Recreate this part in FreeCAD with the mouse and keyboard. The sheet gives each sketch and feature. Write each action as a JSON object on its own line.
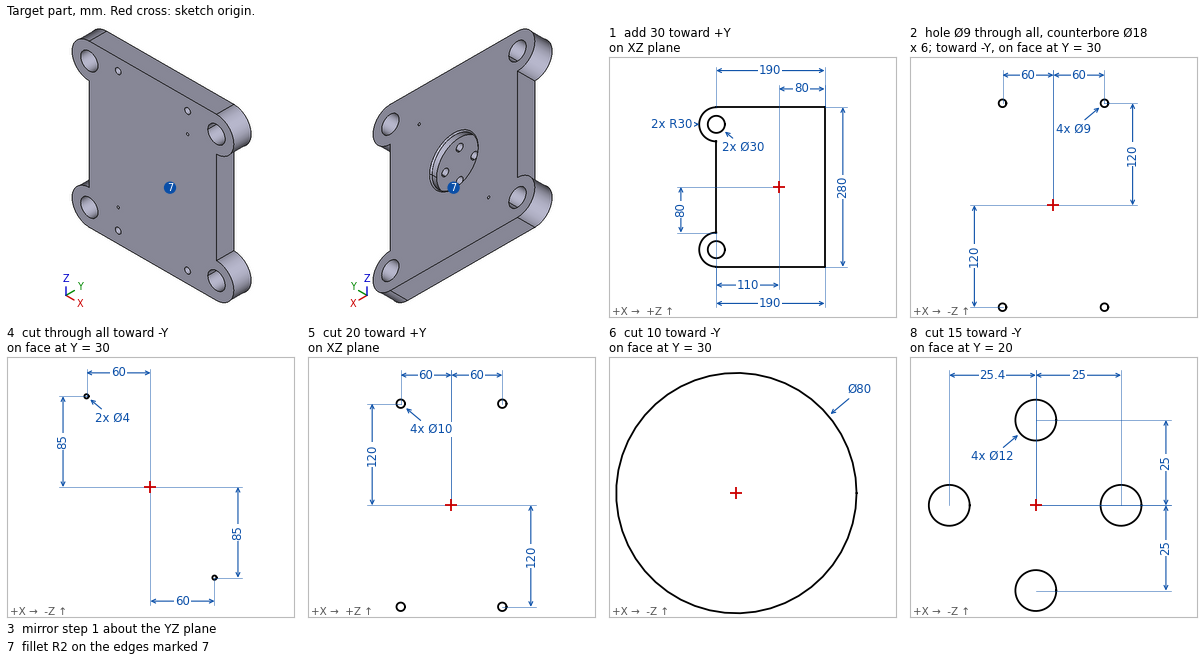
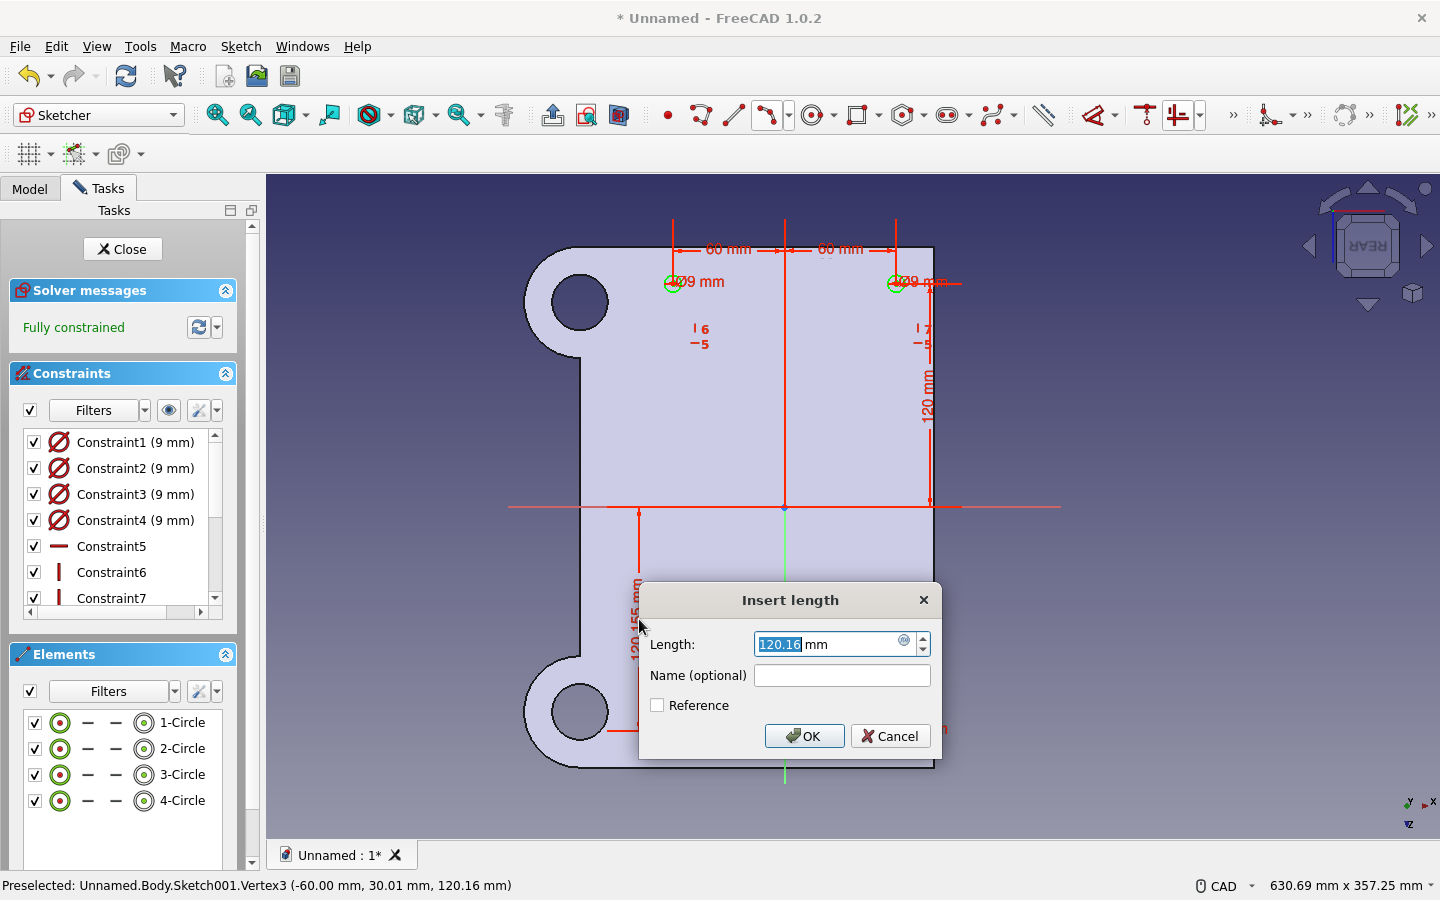
{"action": "type", "text": "120"}
{"action": "key", "text": "Return"}
{"action": "key", "text": "Escape"}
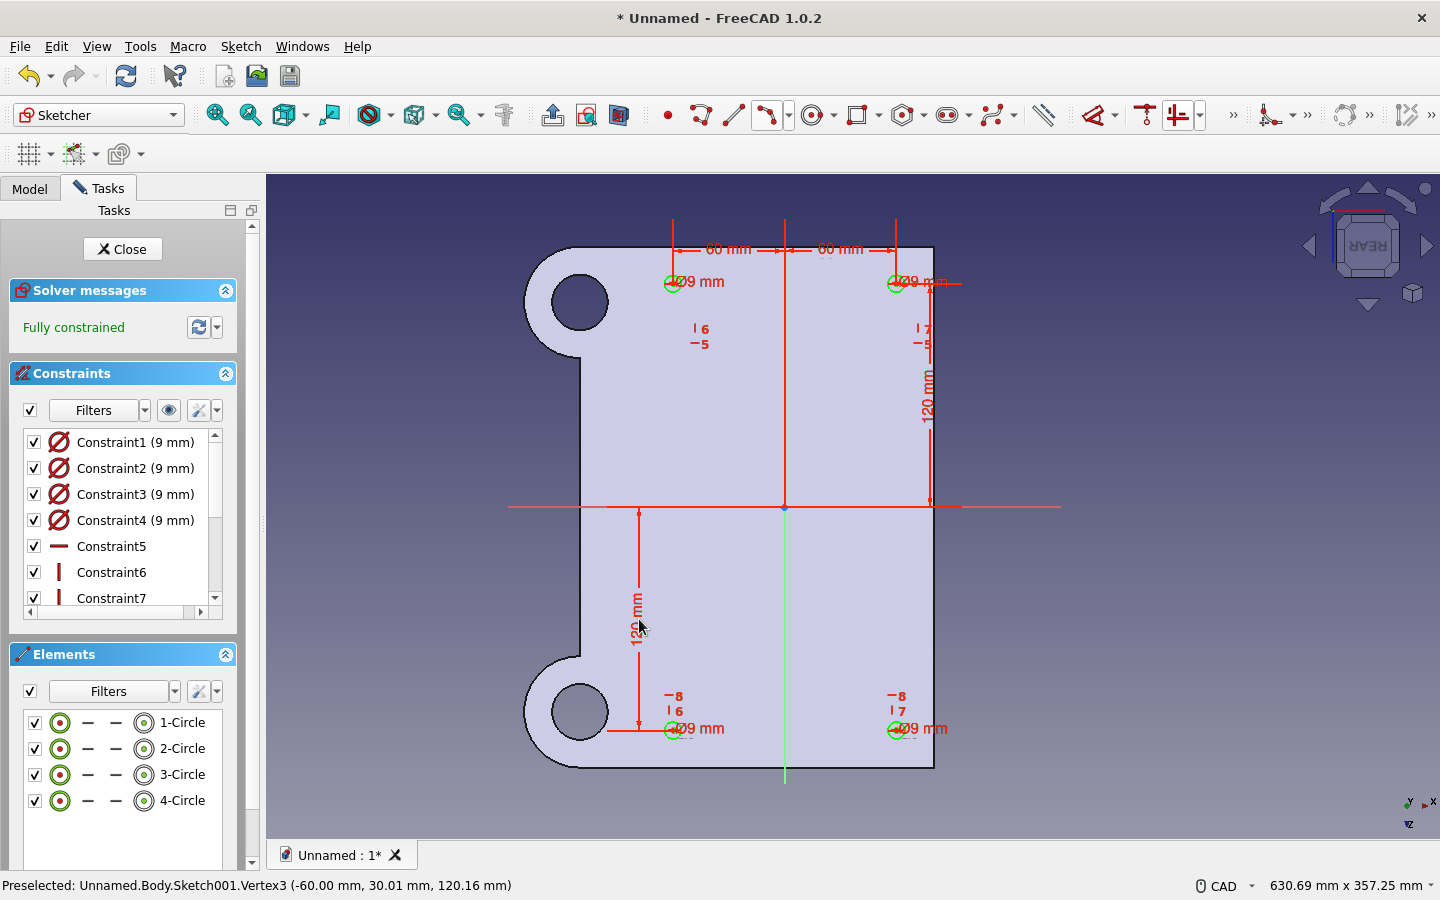
{"action": "left_click", "coordinate": [123, 249]}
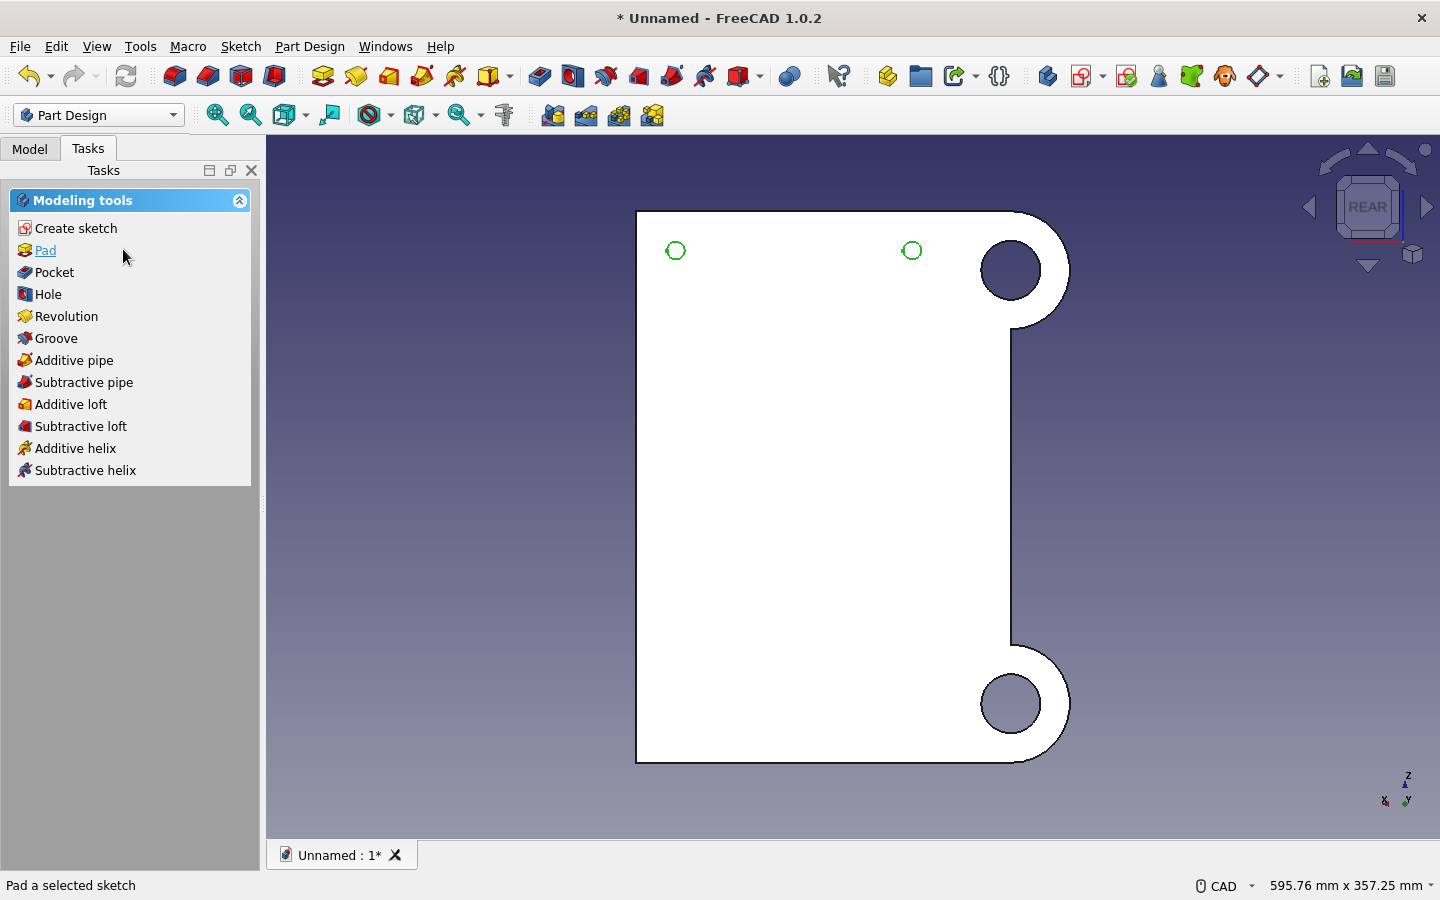
{"action": "left_click", "coordinate": [573, 76]}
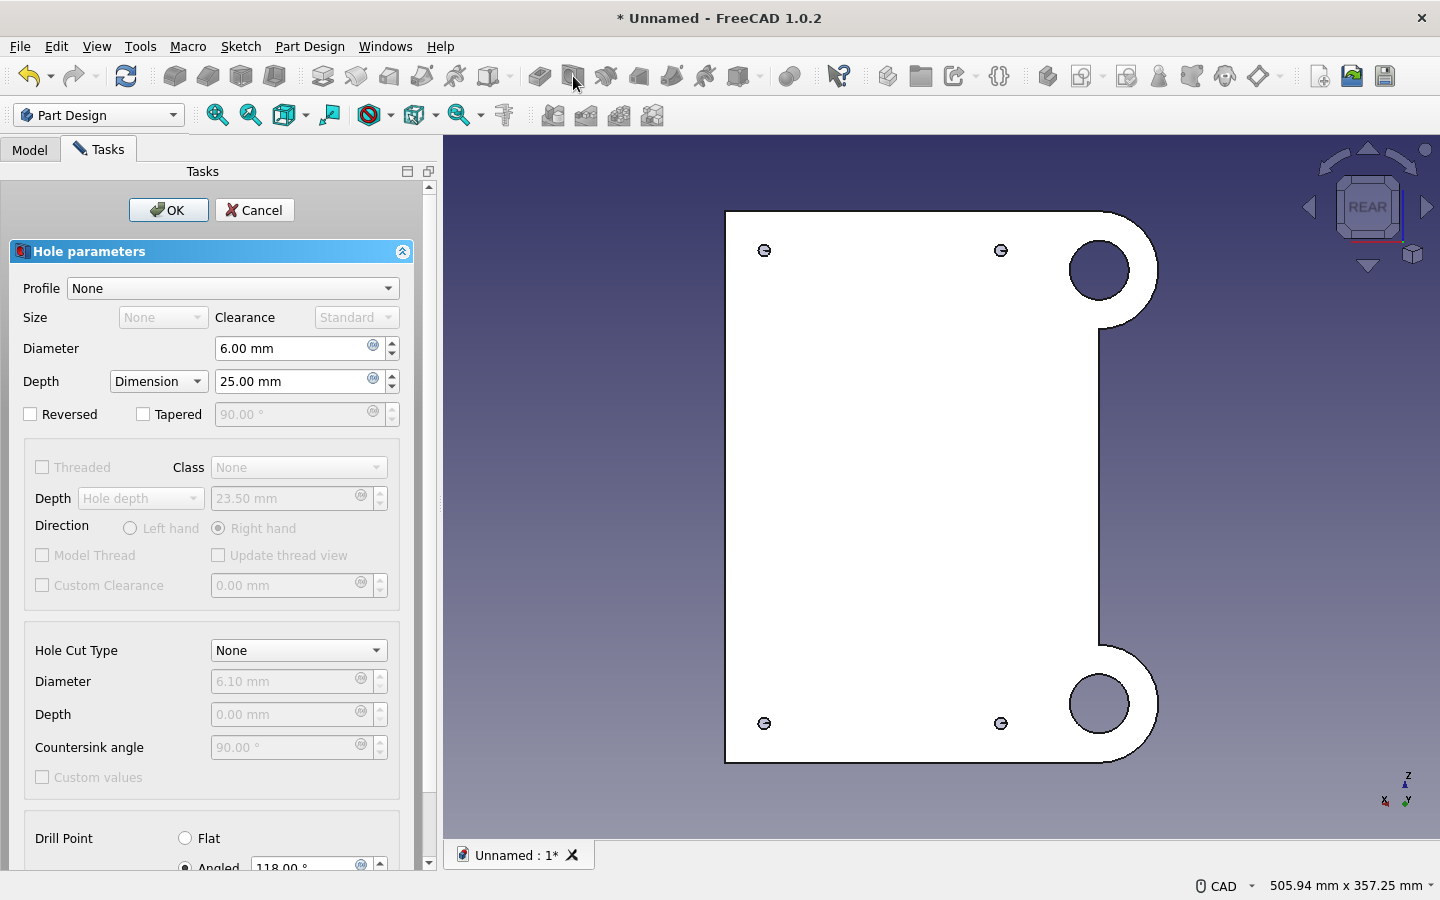
{"action": "triple_click", "coordinate": [300, 348]}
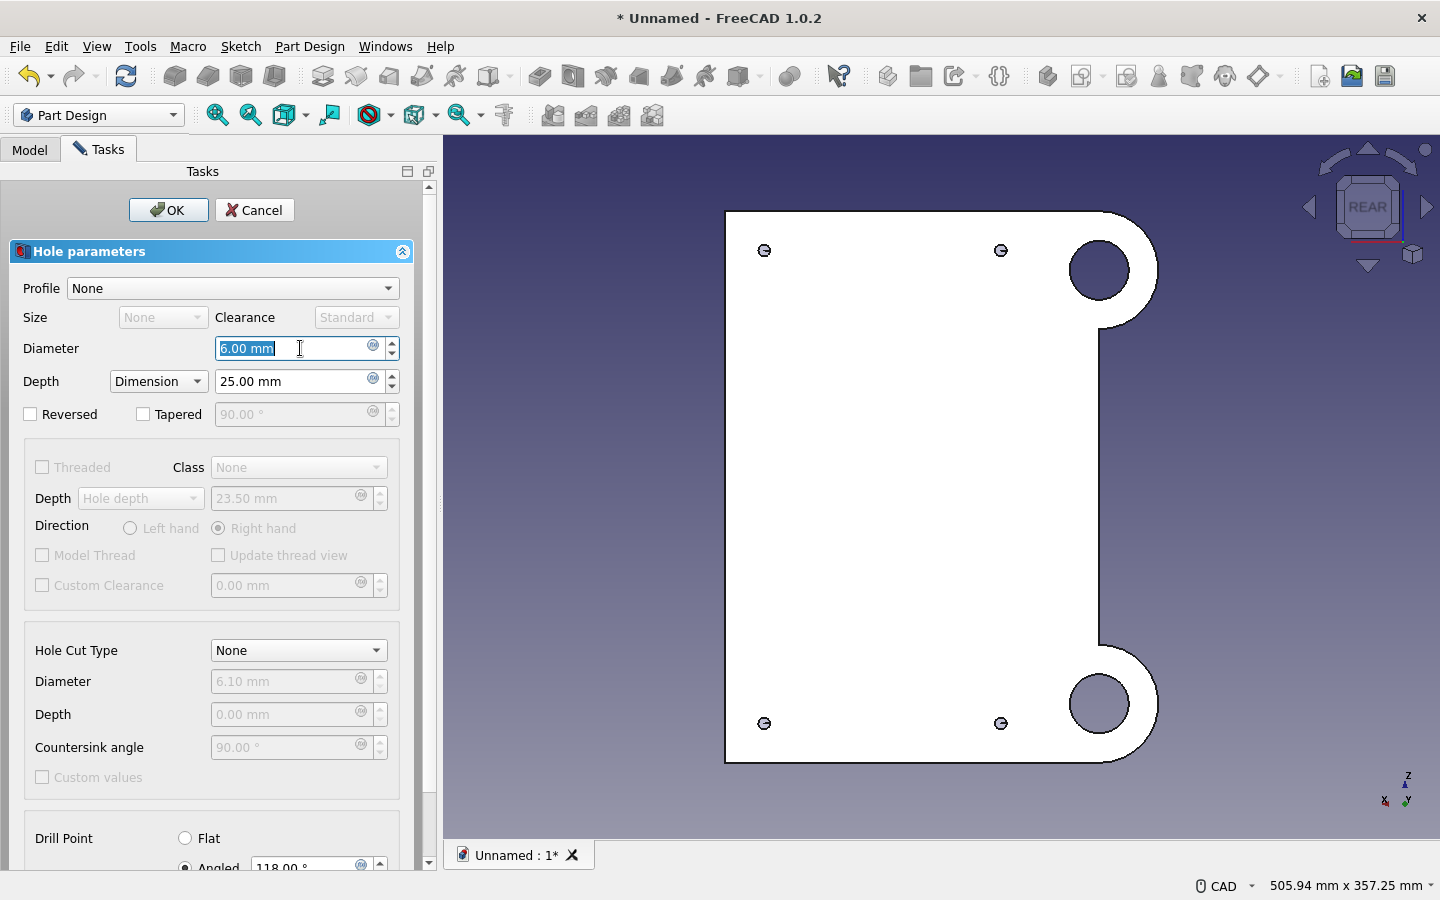
{"action": "type", "text": "9"}
{"action": "key", "text": "Tab"}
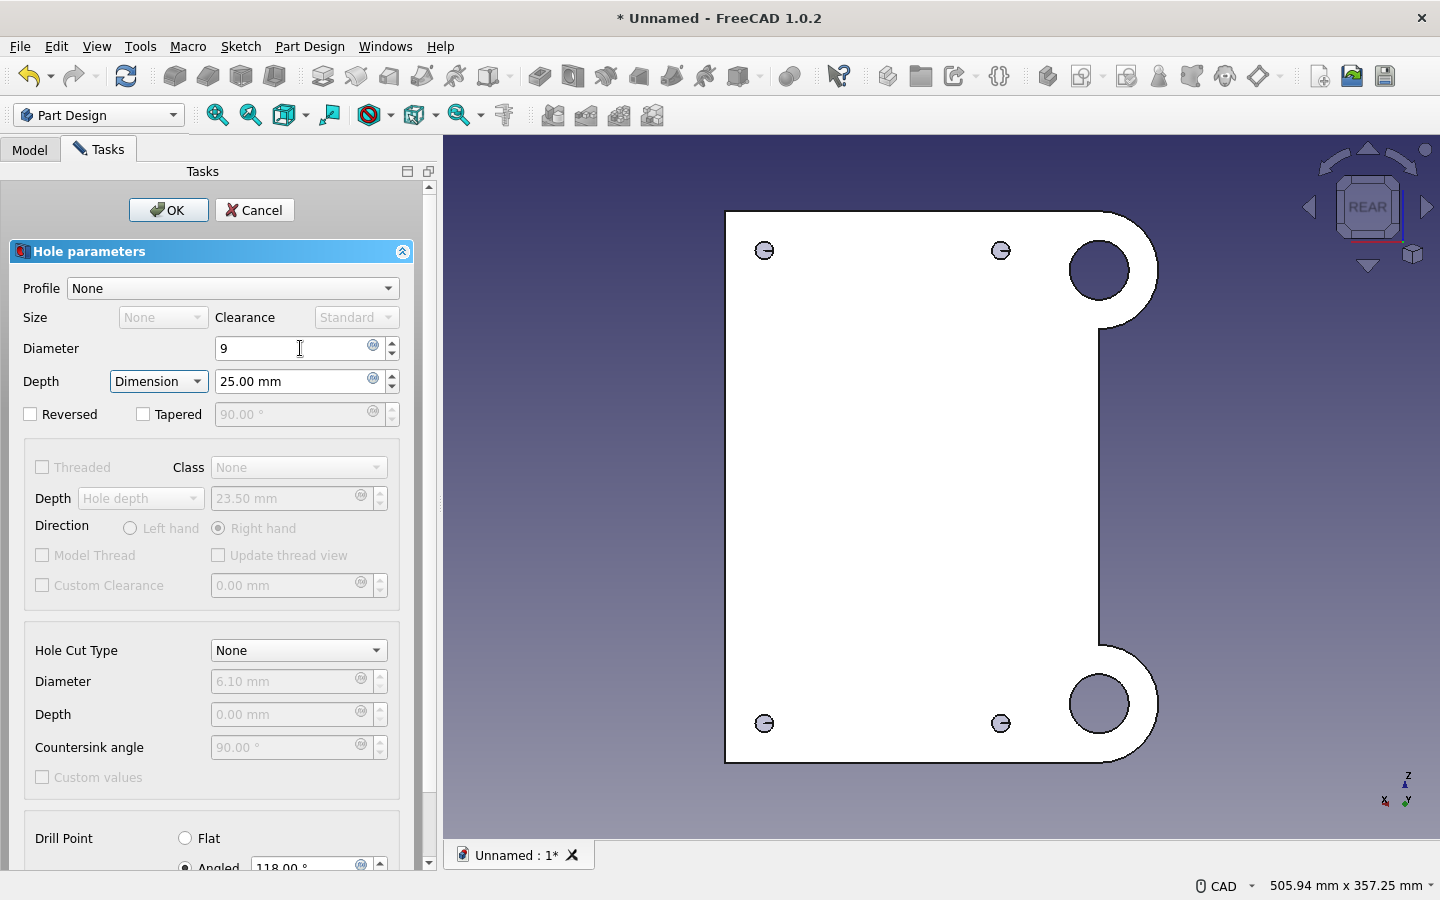
{"action": "left_click", "coordinate": [160, 382]}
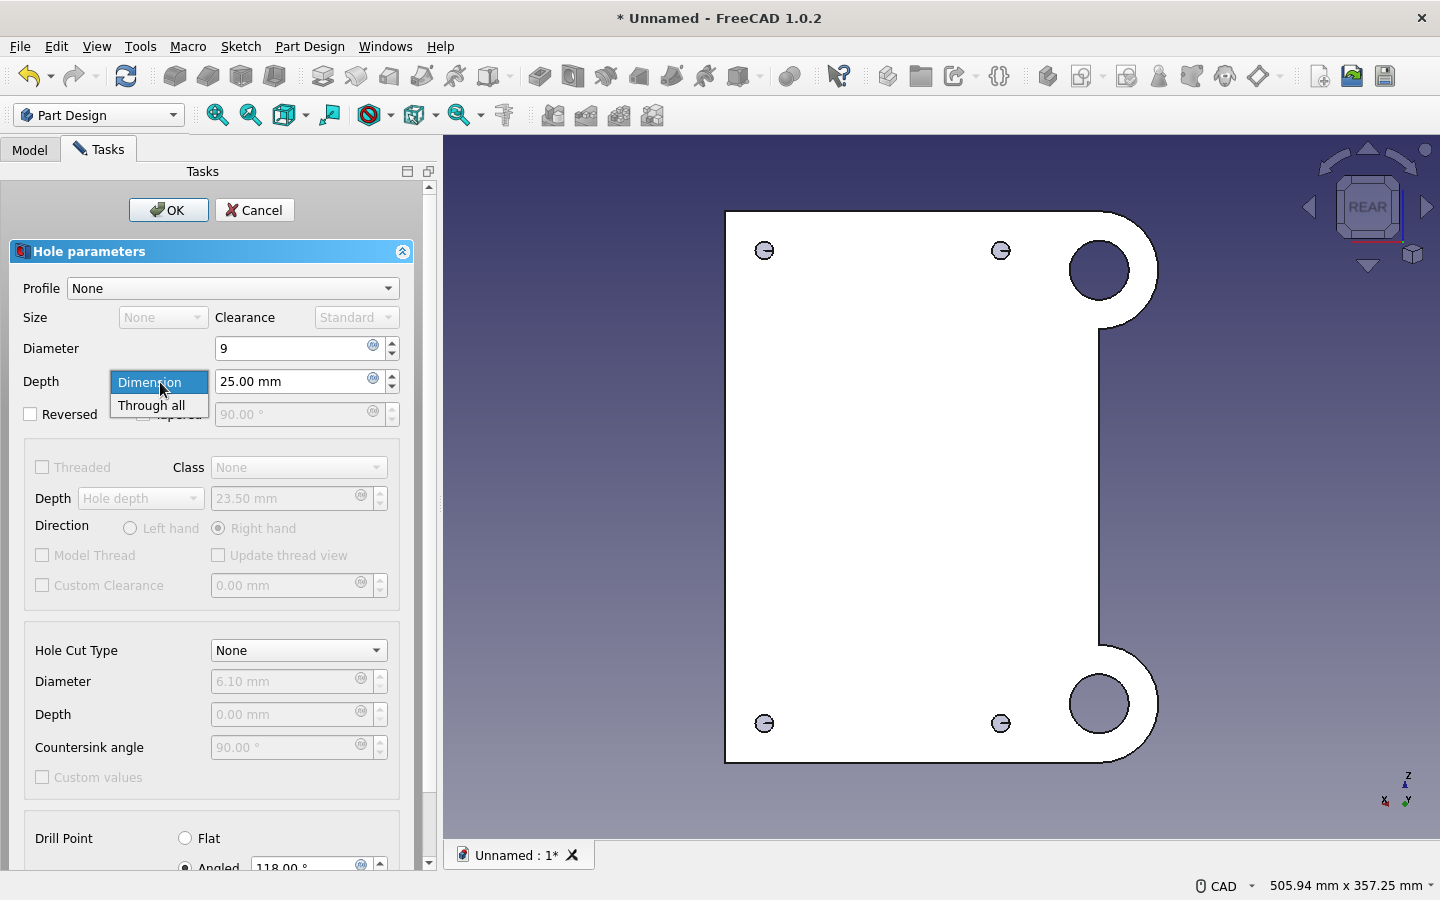
{"action": "left_click", "coordinate": [158, 406]}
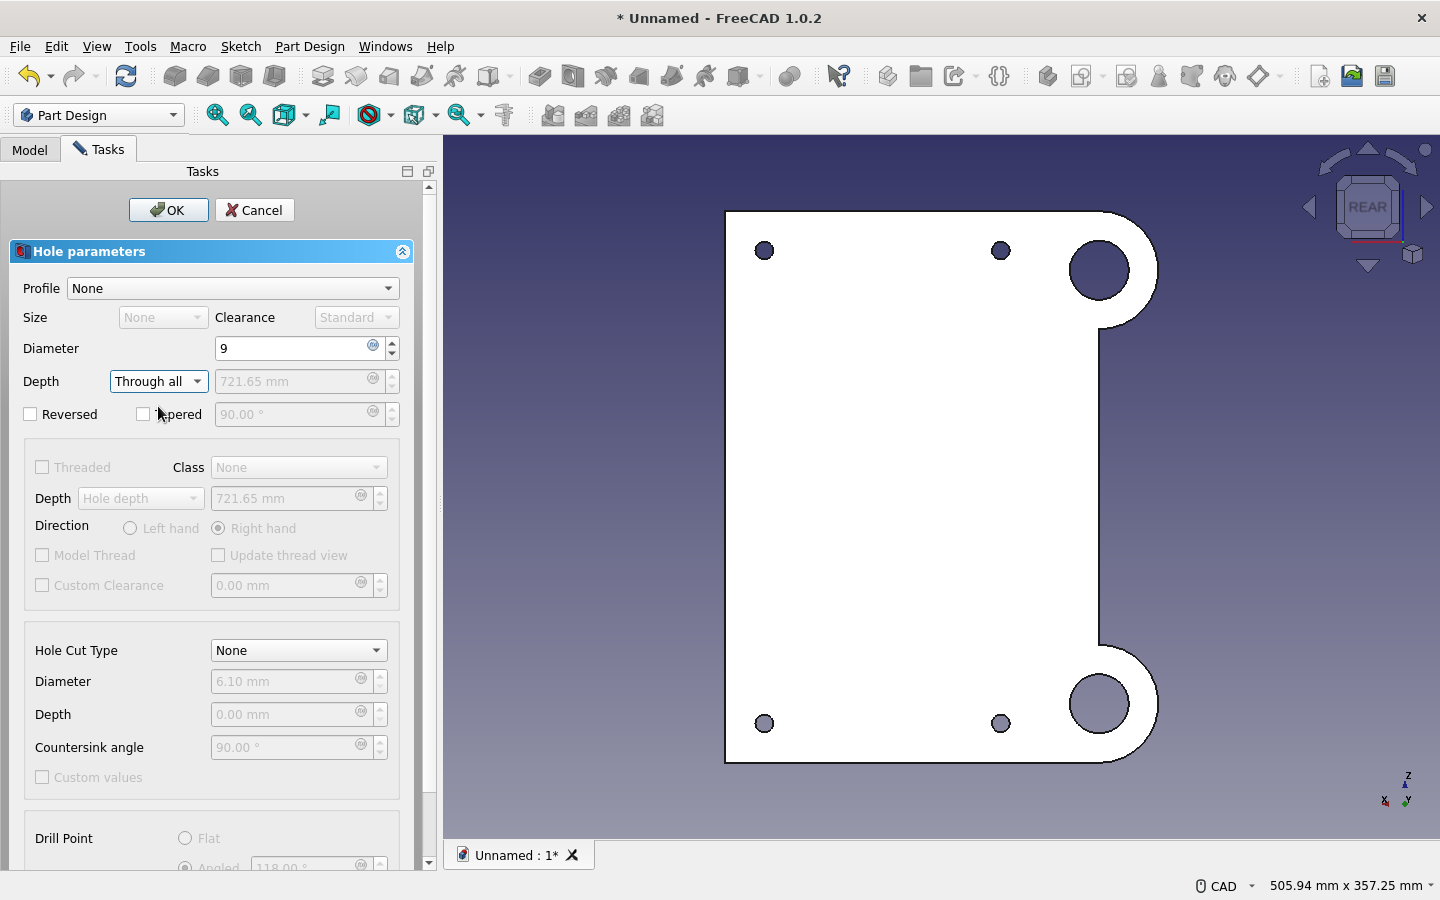
{"action": "left_click", "coordinate": [300, 650]}